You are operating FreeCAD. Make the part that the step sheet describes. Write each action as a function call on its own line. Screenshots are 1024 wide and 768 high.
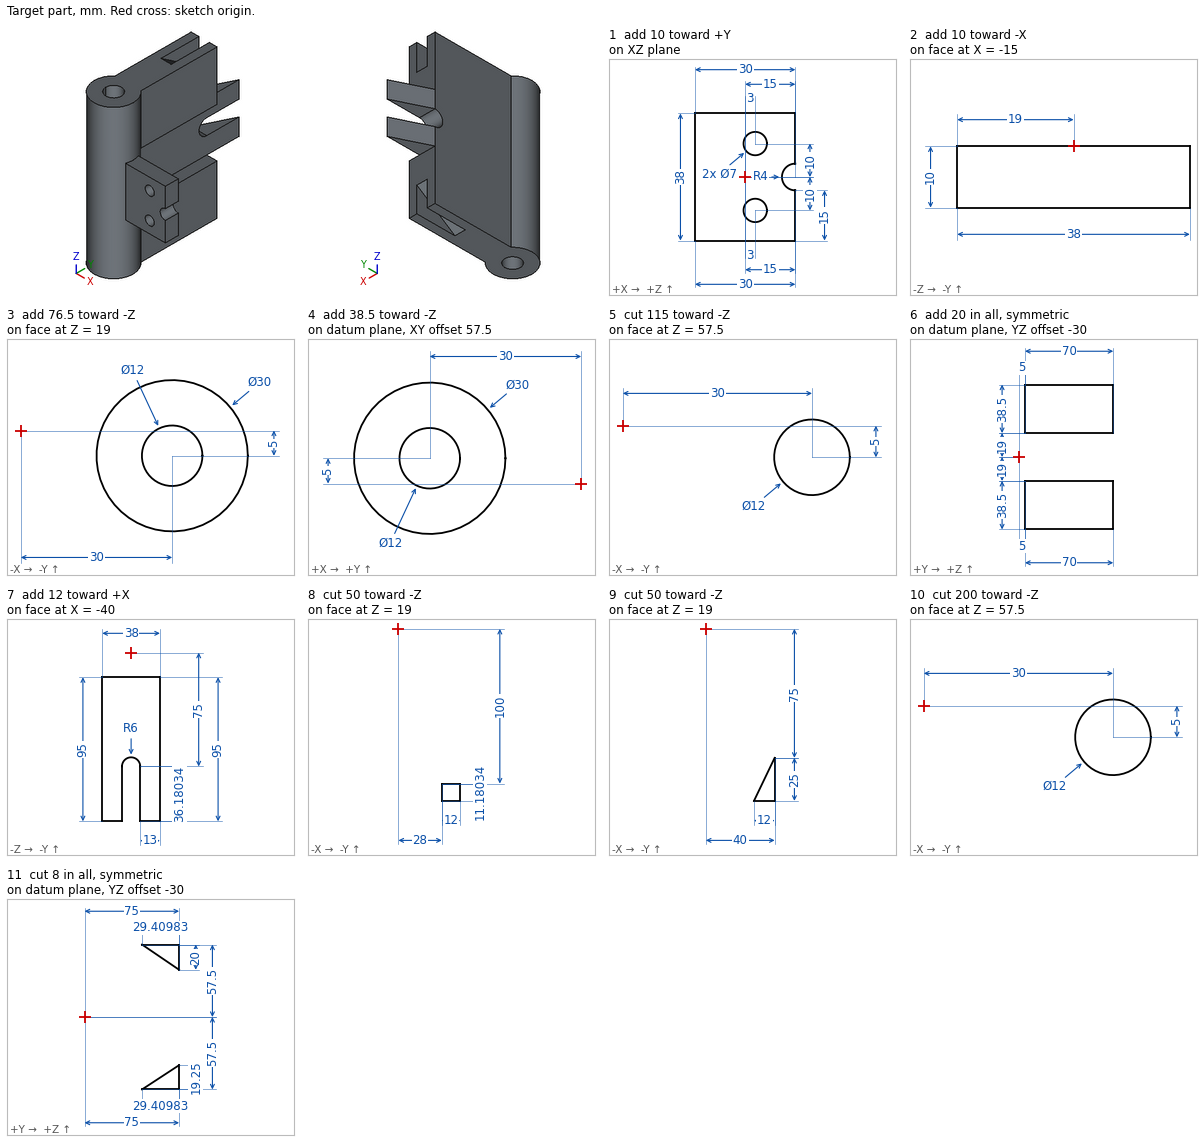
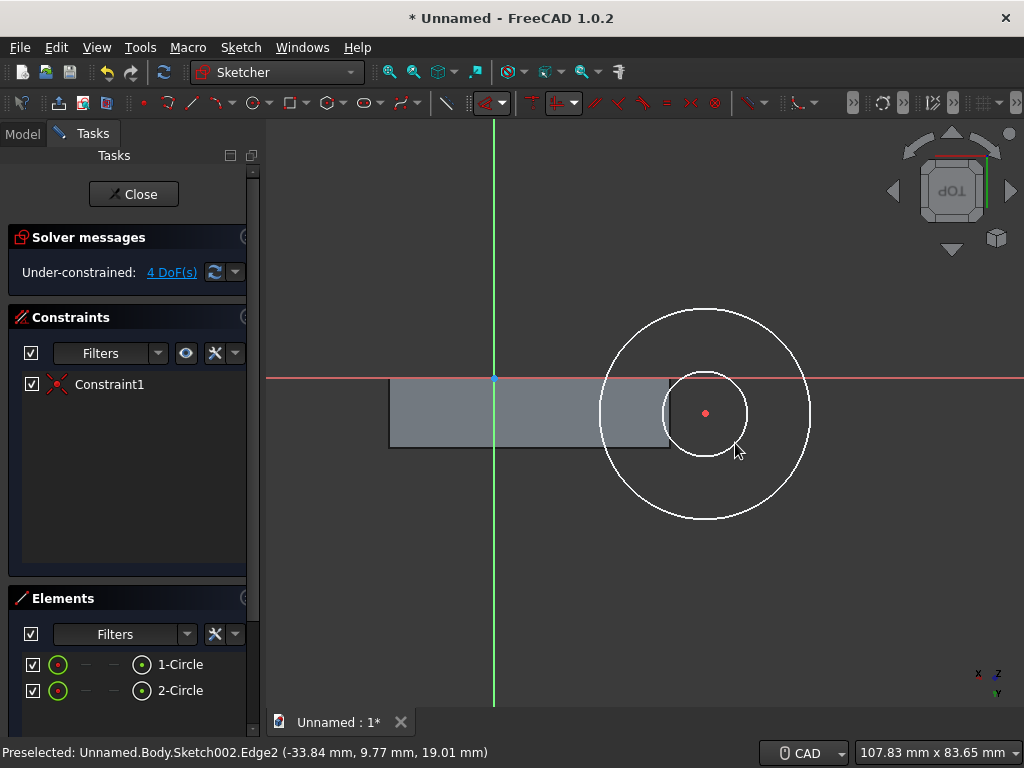
click(779, 339)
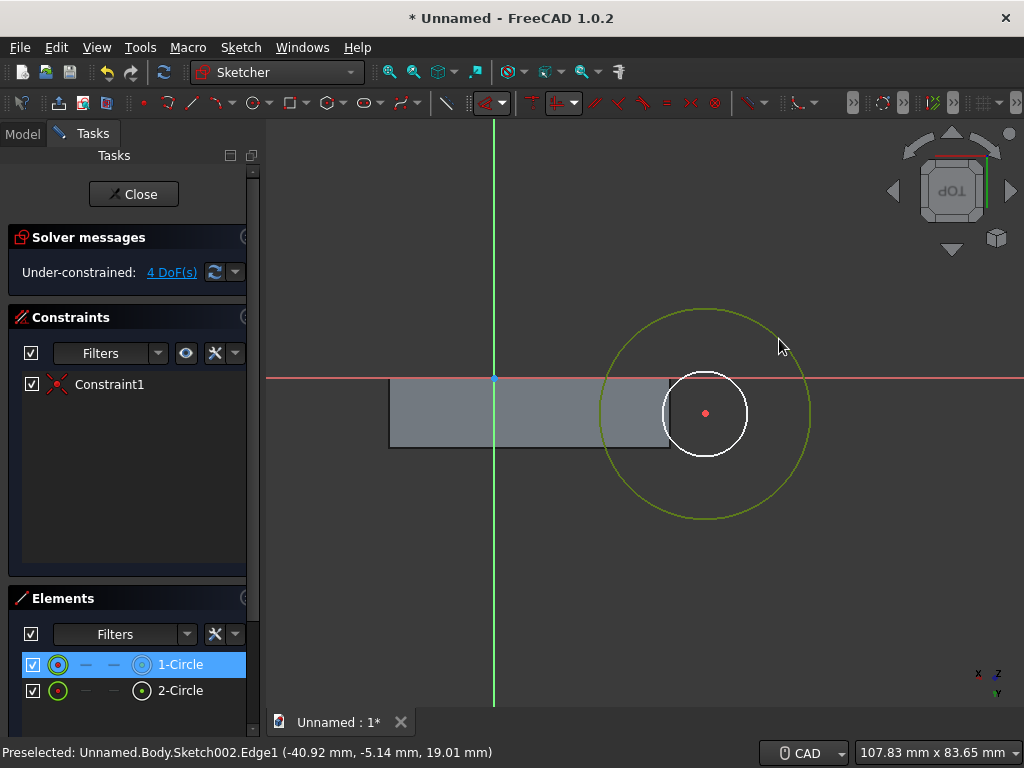
key(k)
key(o)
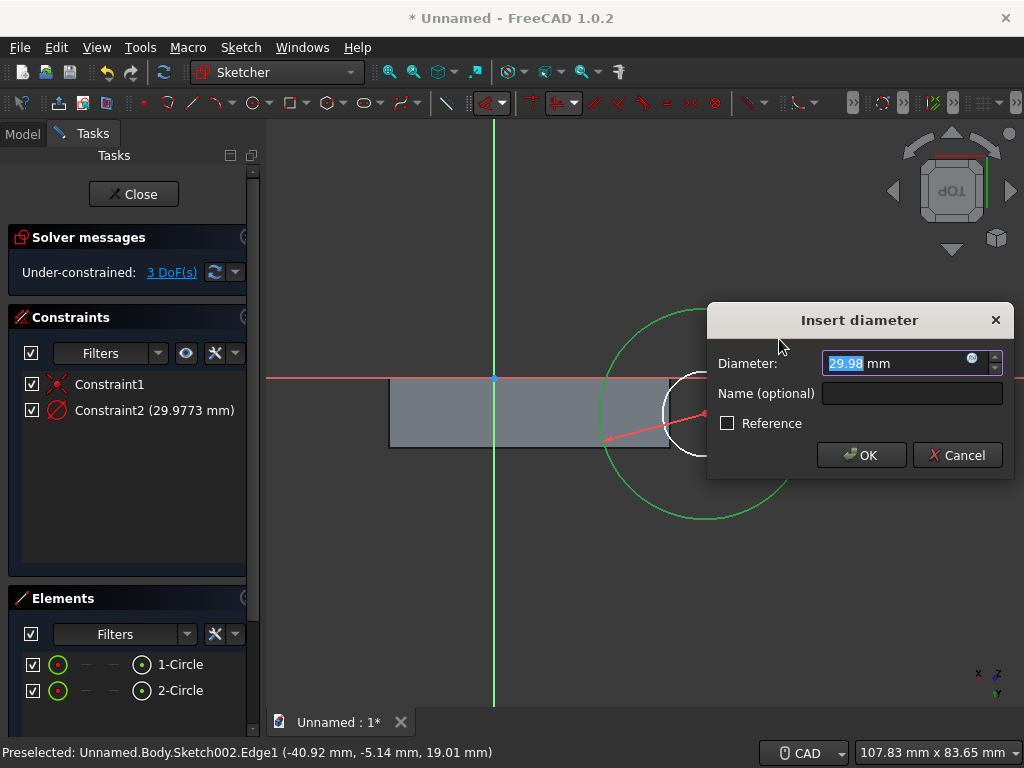
text(30)
key(Return)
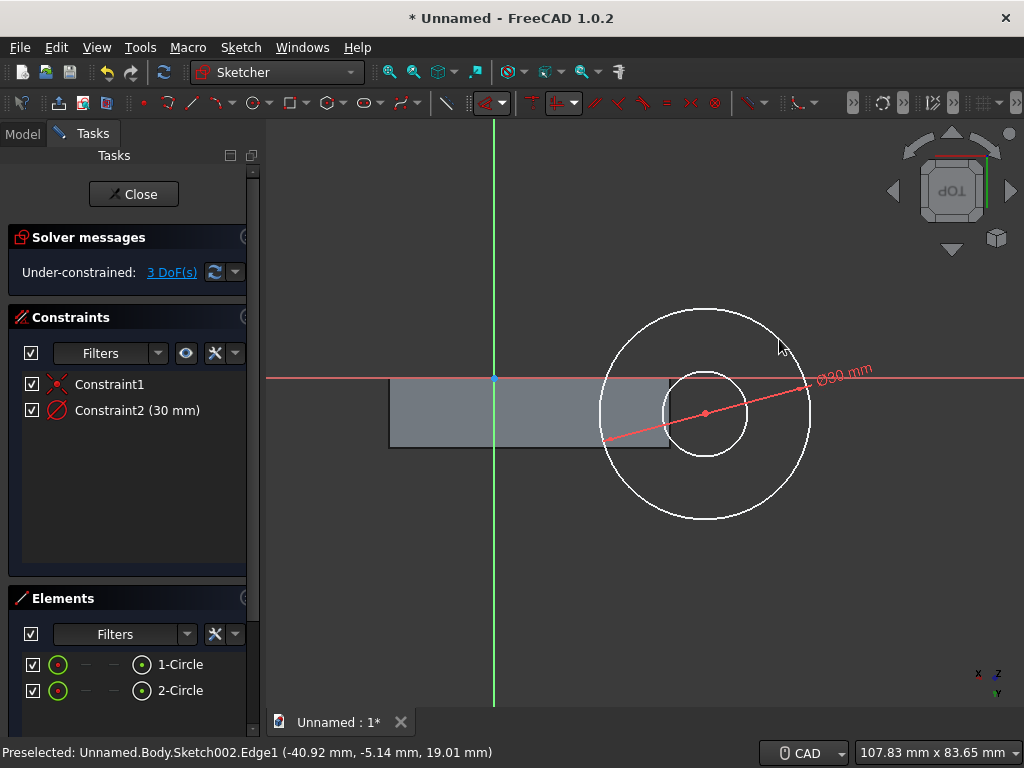
click(675, 444)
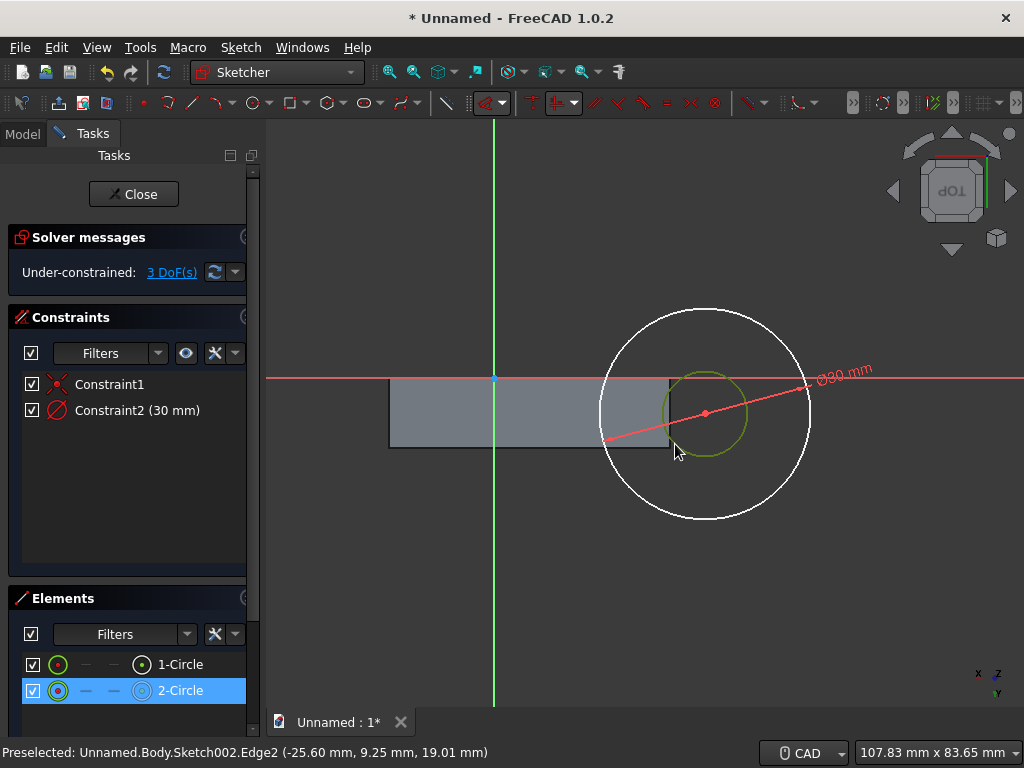
key(k)
key(o)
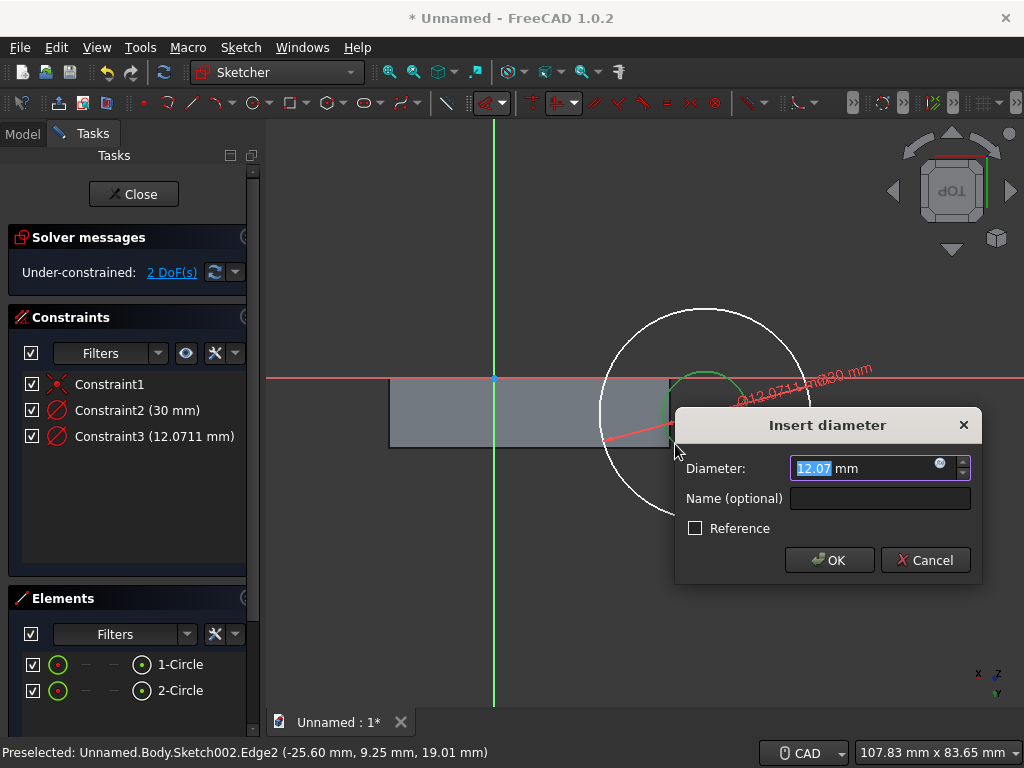
text(12)
key(Return)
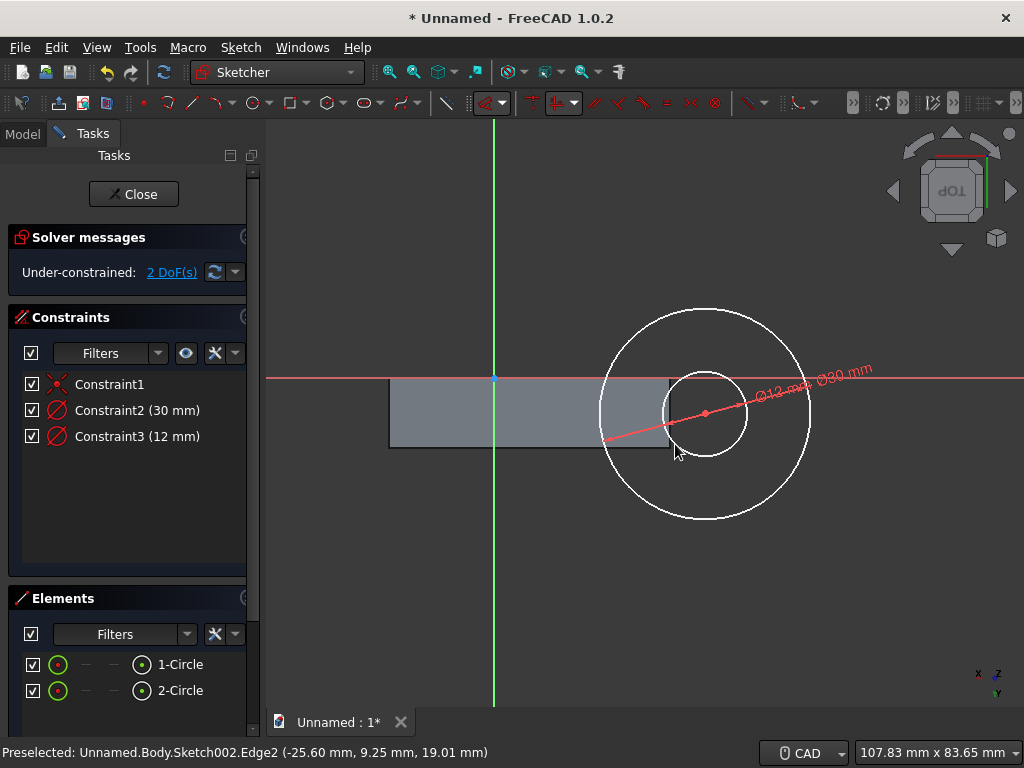
click(705, 414)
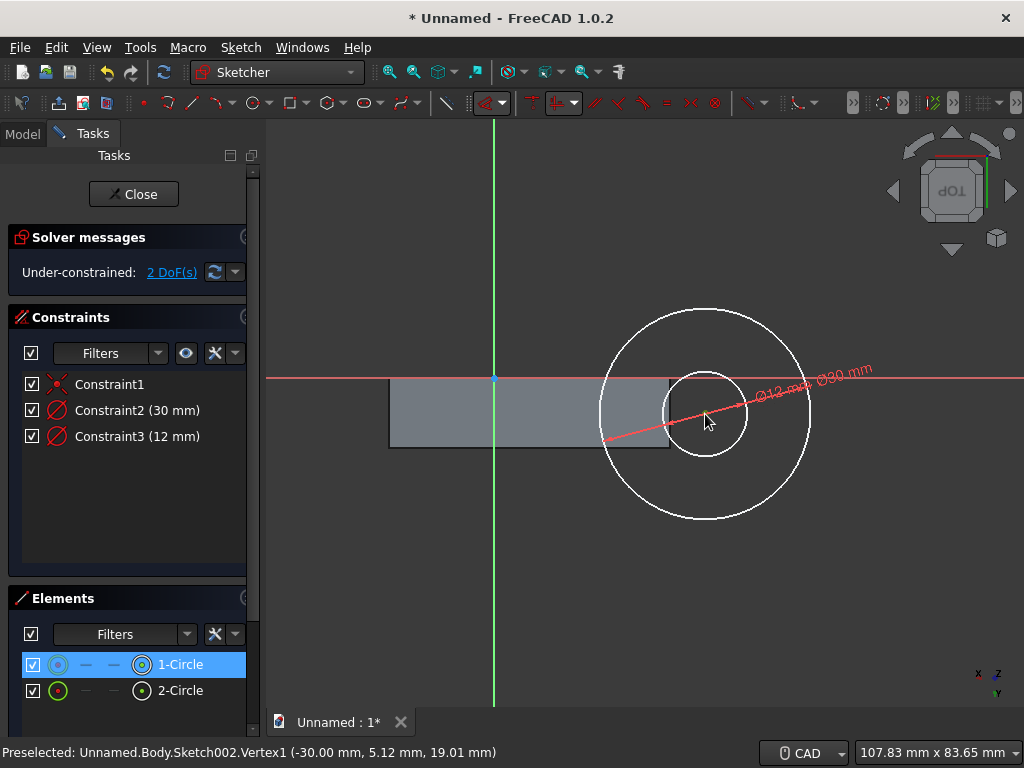
click(504, 104)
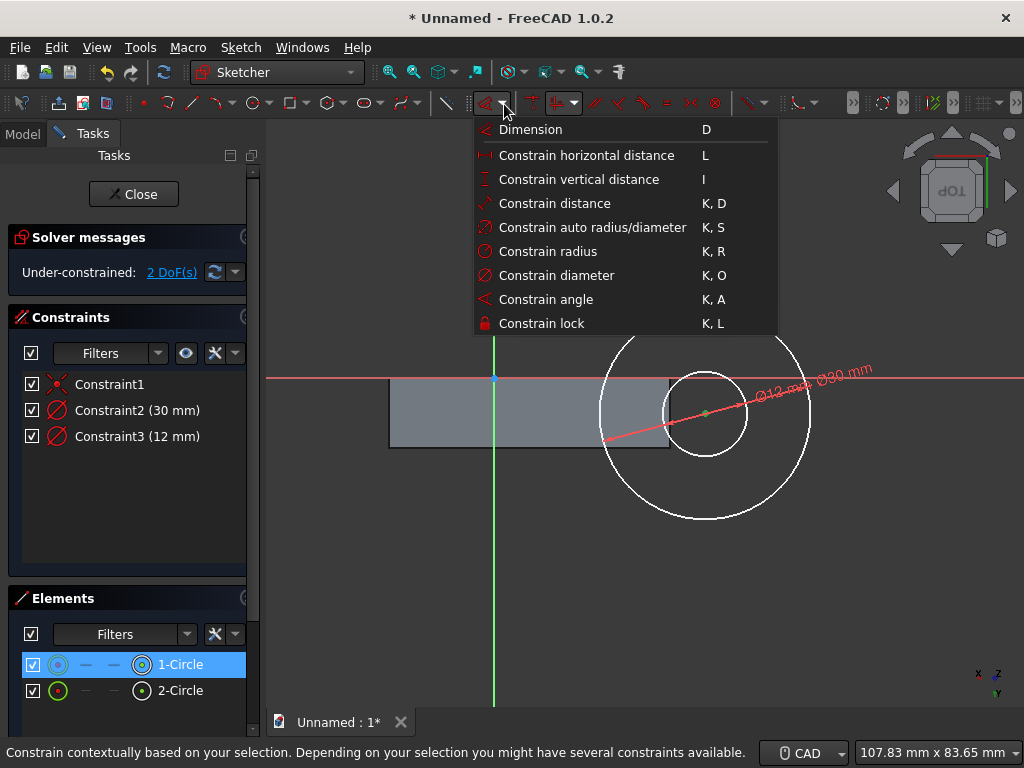
click(626, 179)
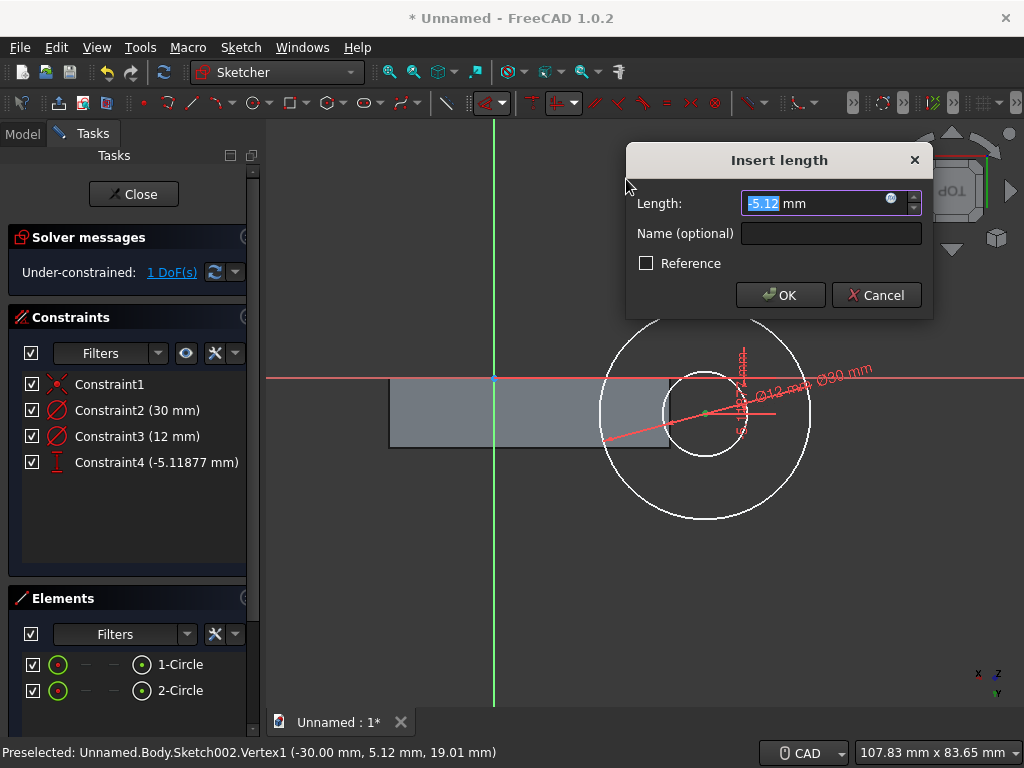
text(-5)
key(Return)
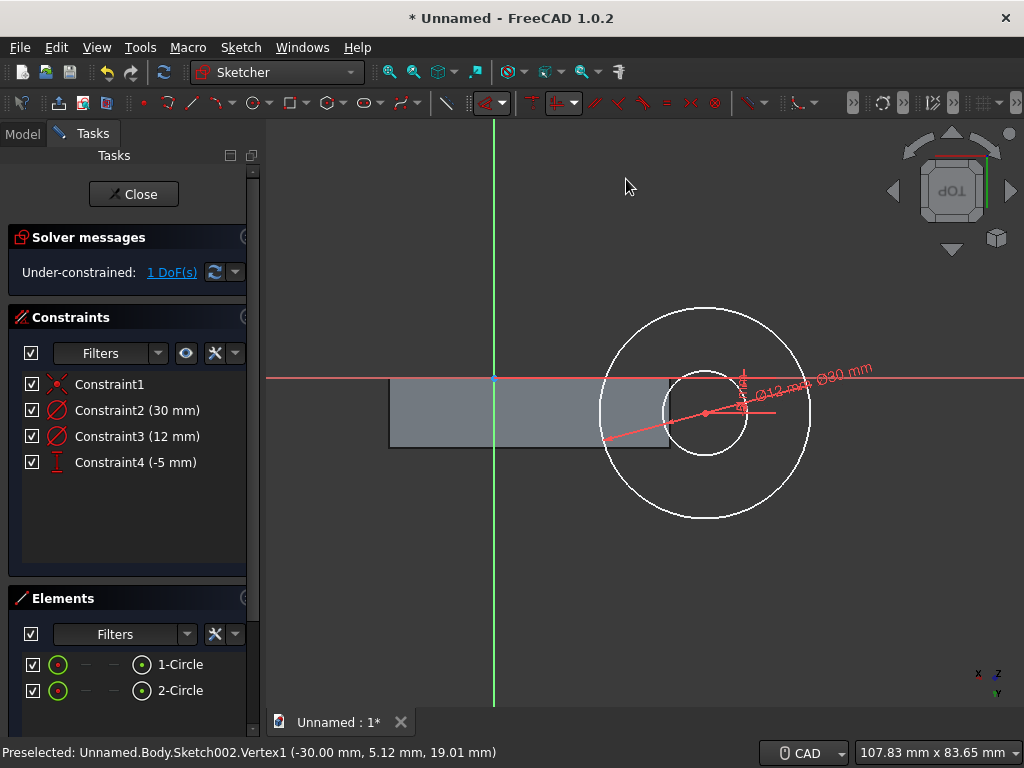
click(705, 413)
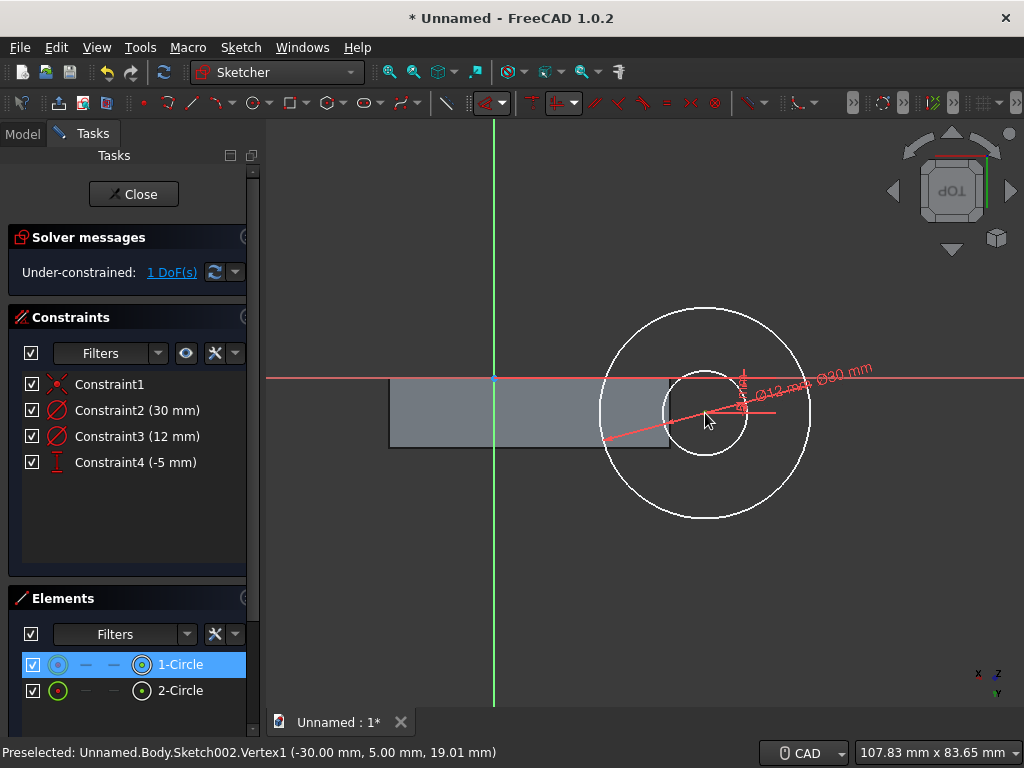
key(l)